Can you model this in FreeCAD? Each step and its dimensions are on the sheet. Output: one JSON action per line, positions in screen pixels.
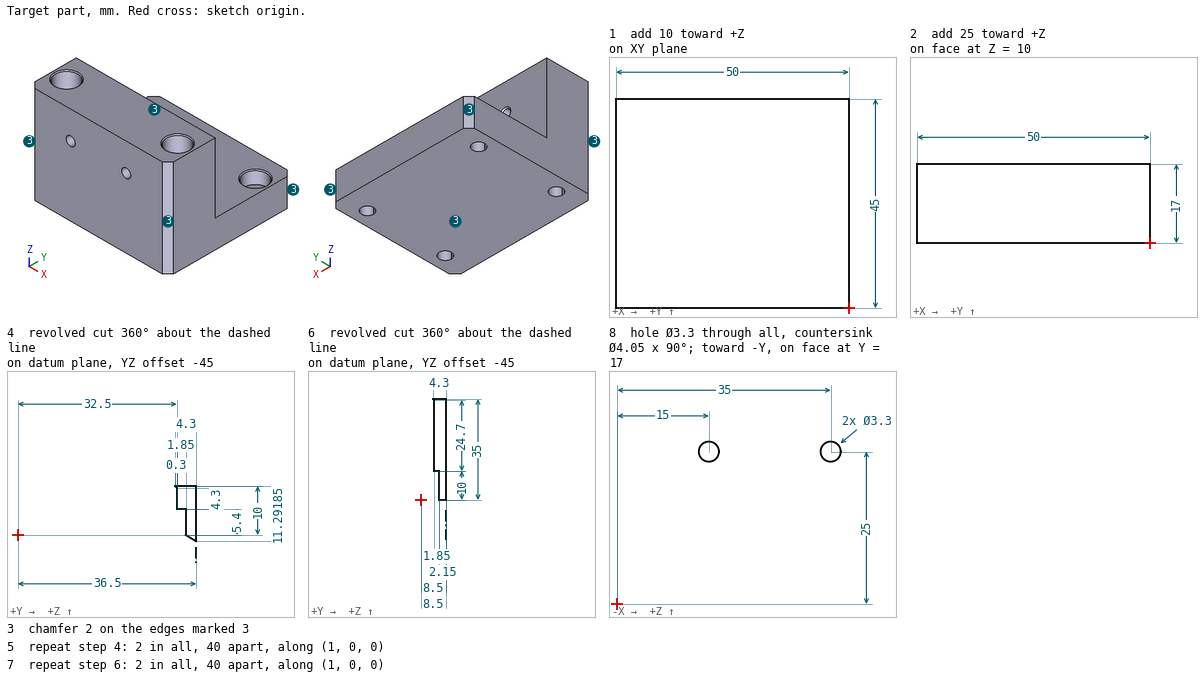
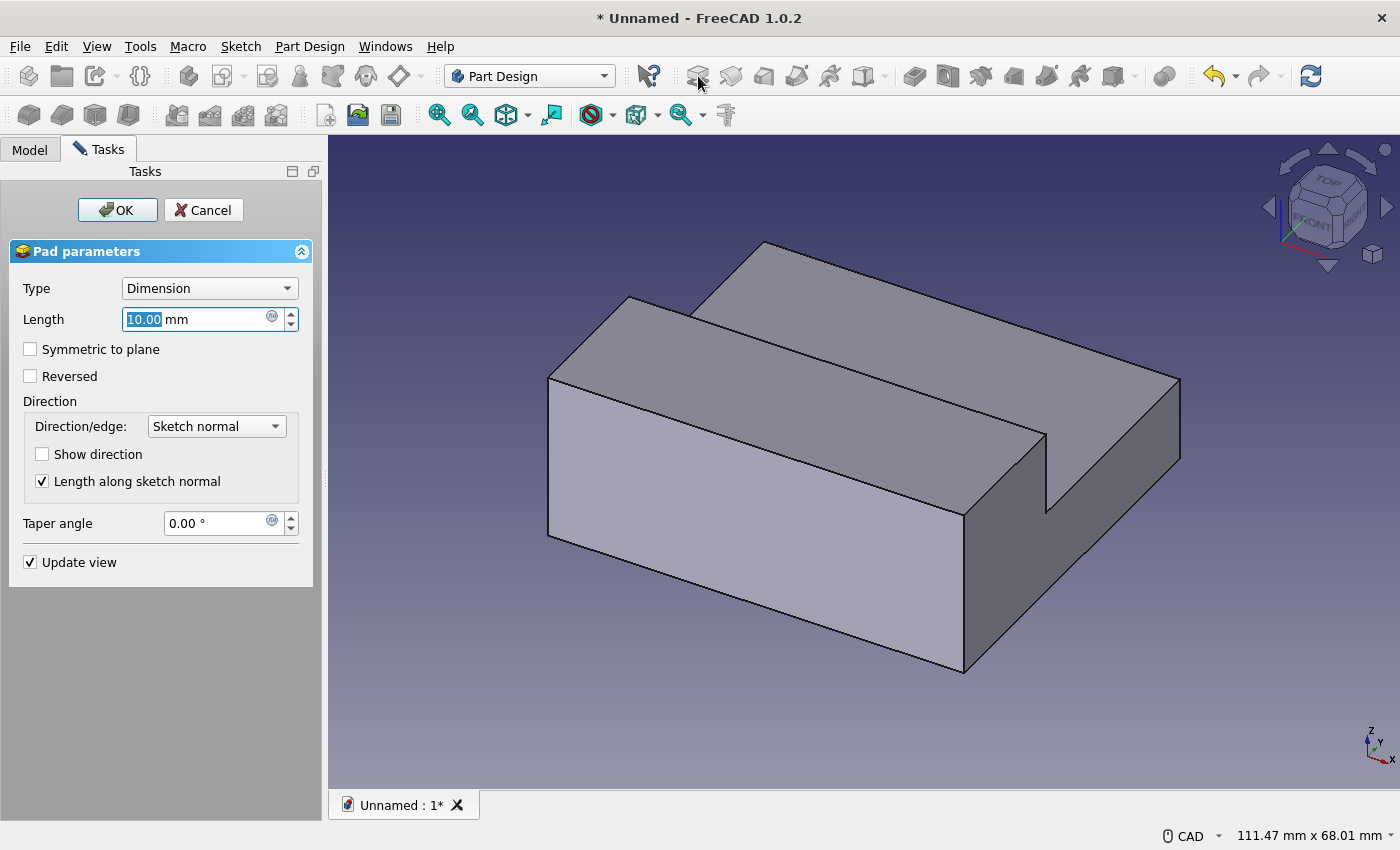
{"action": "type", "text": "25"}
{"action": "key", "text": "Tab"}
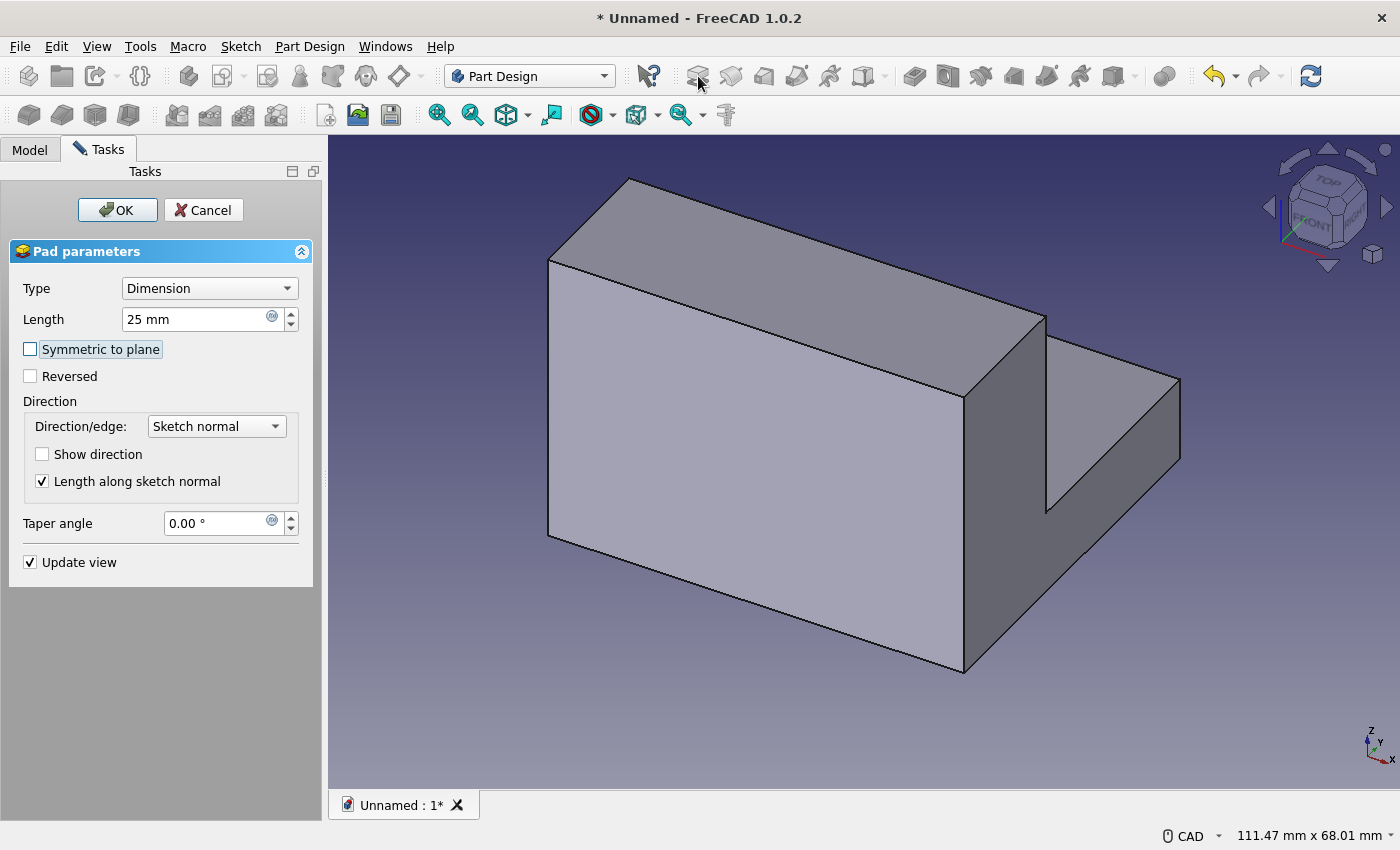
{"action": "left_click", "coordinate": [118, 210]}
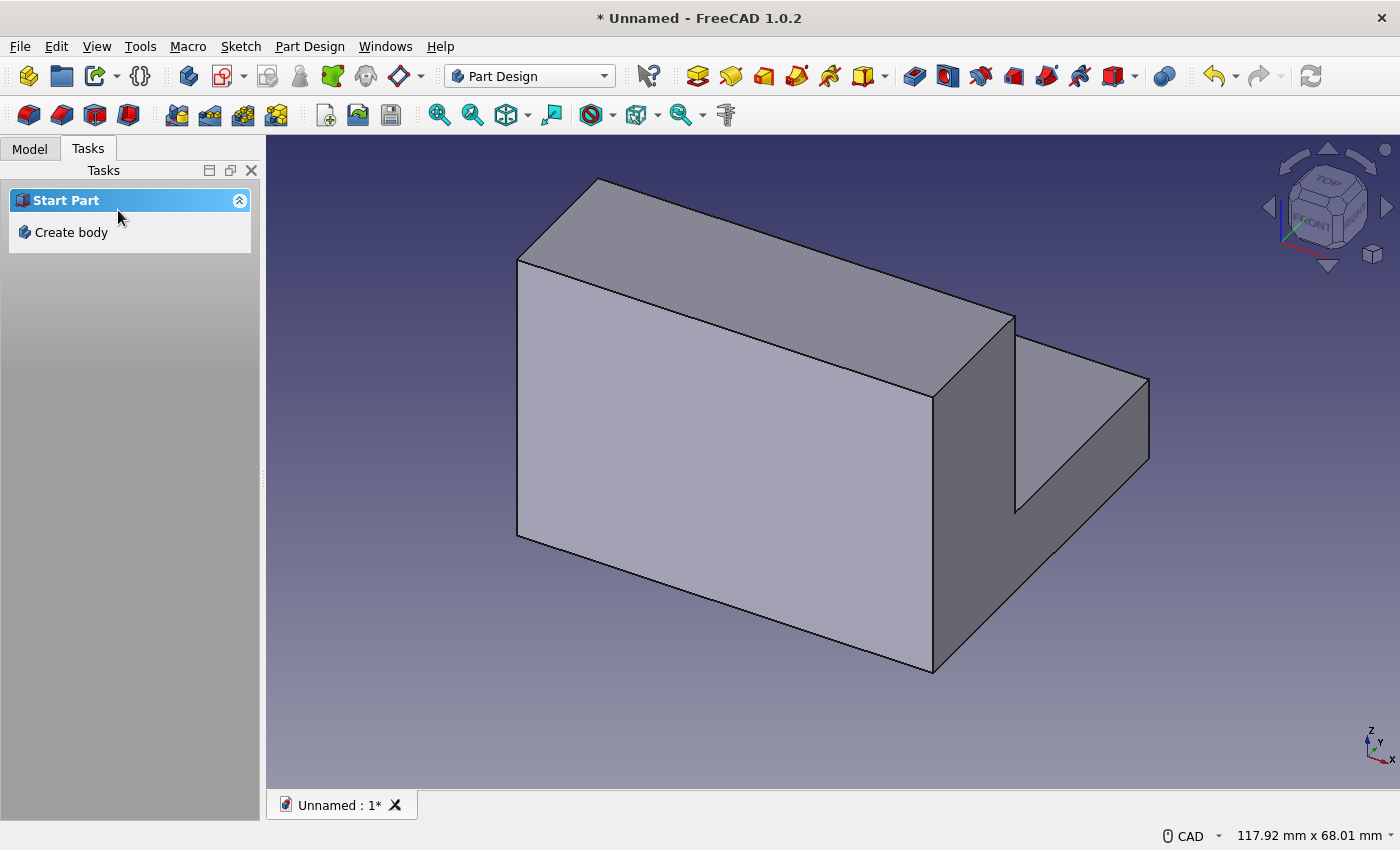
{"action": "key", "text": "v f"}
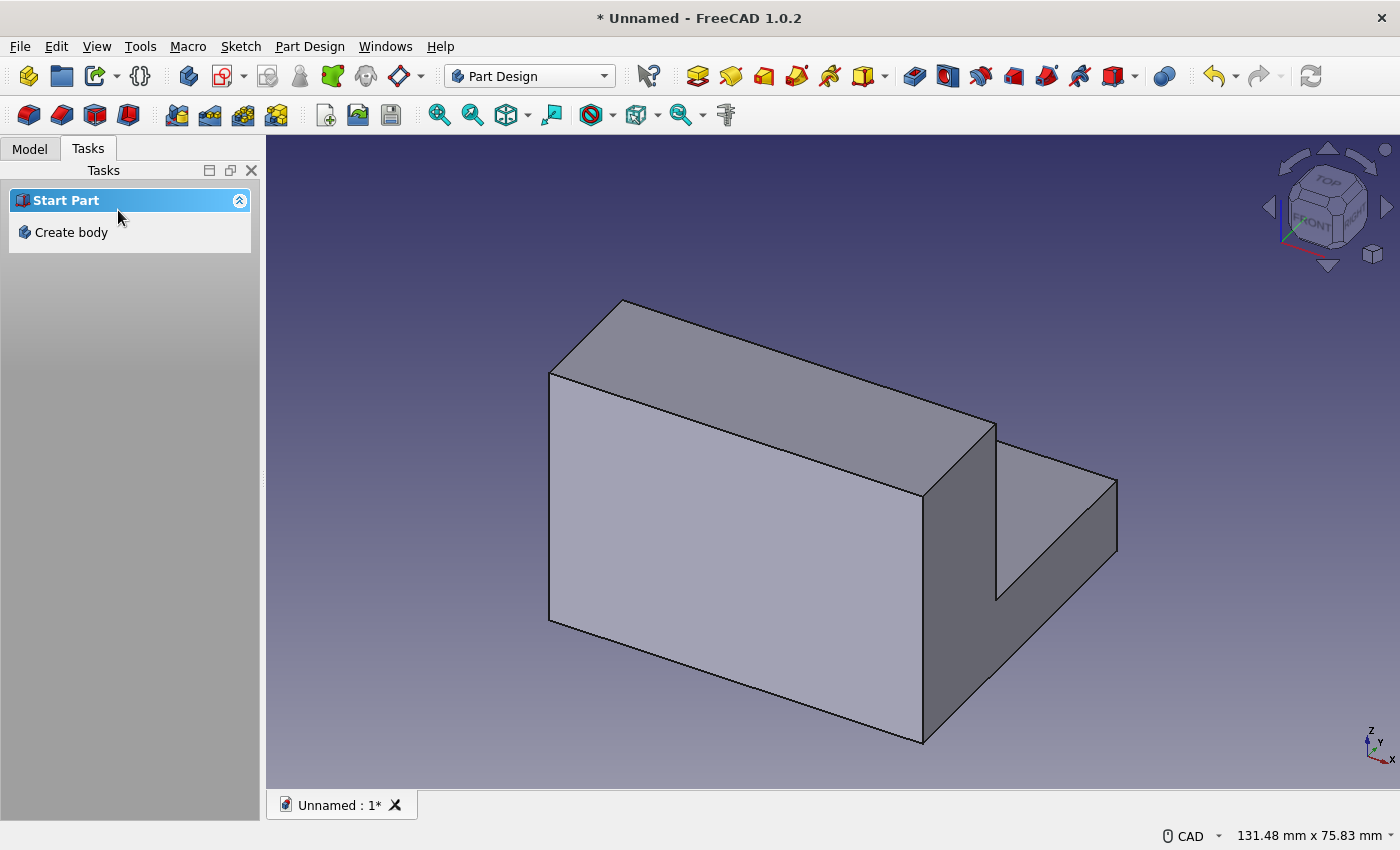
{"action": "left_click", "coordinate": [923, 619]}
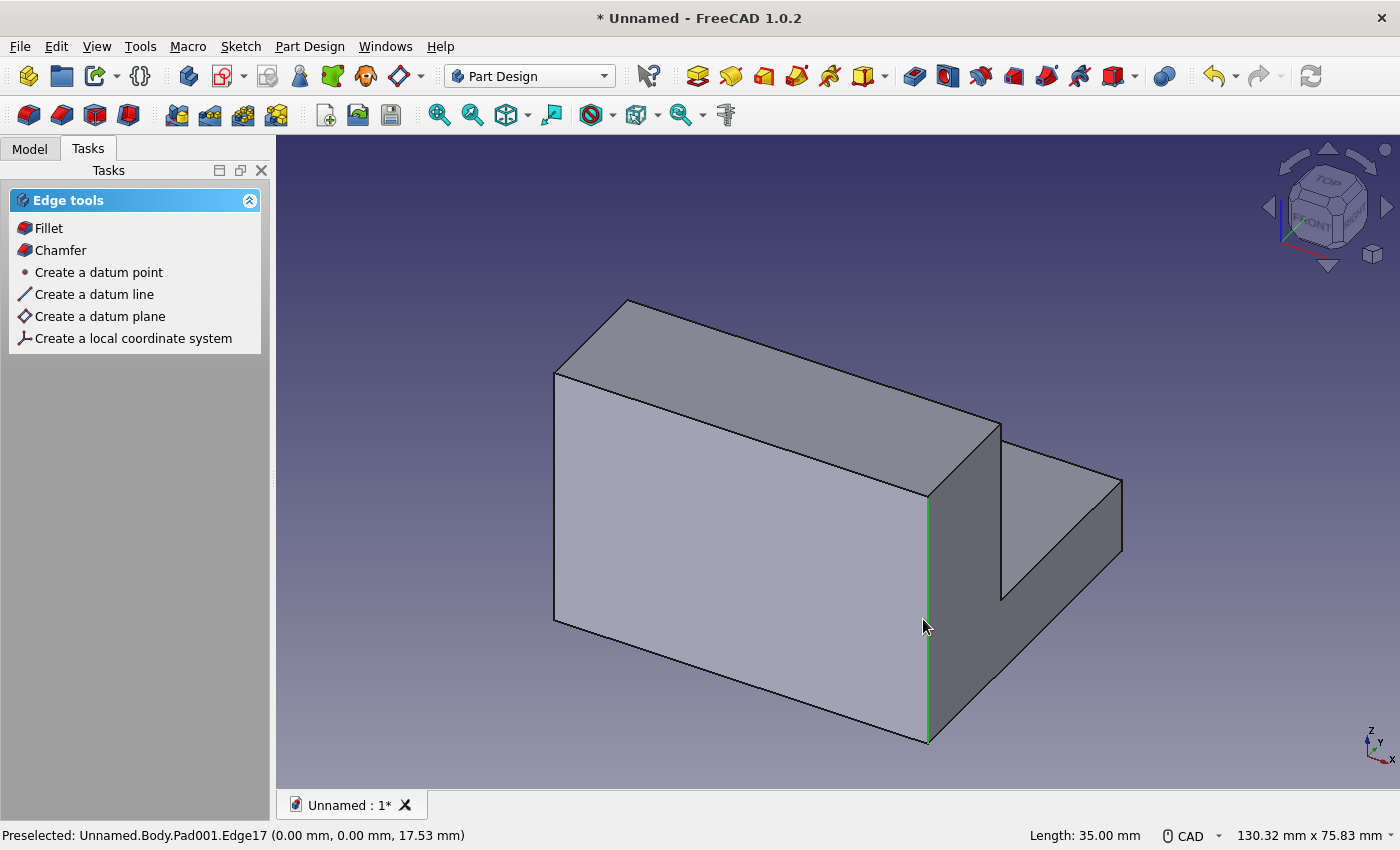
{"action": "key", "text": "0"}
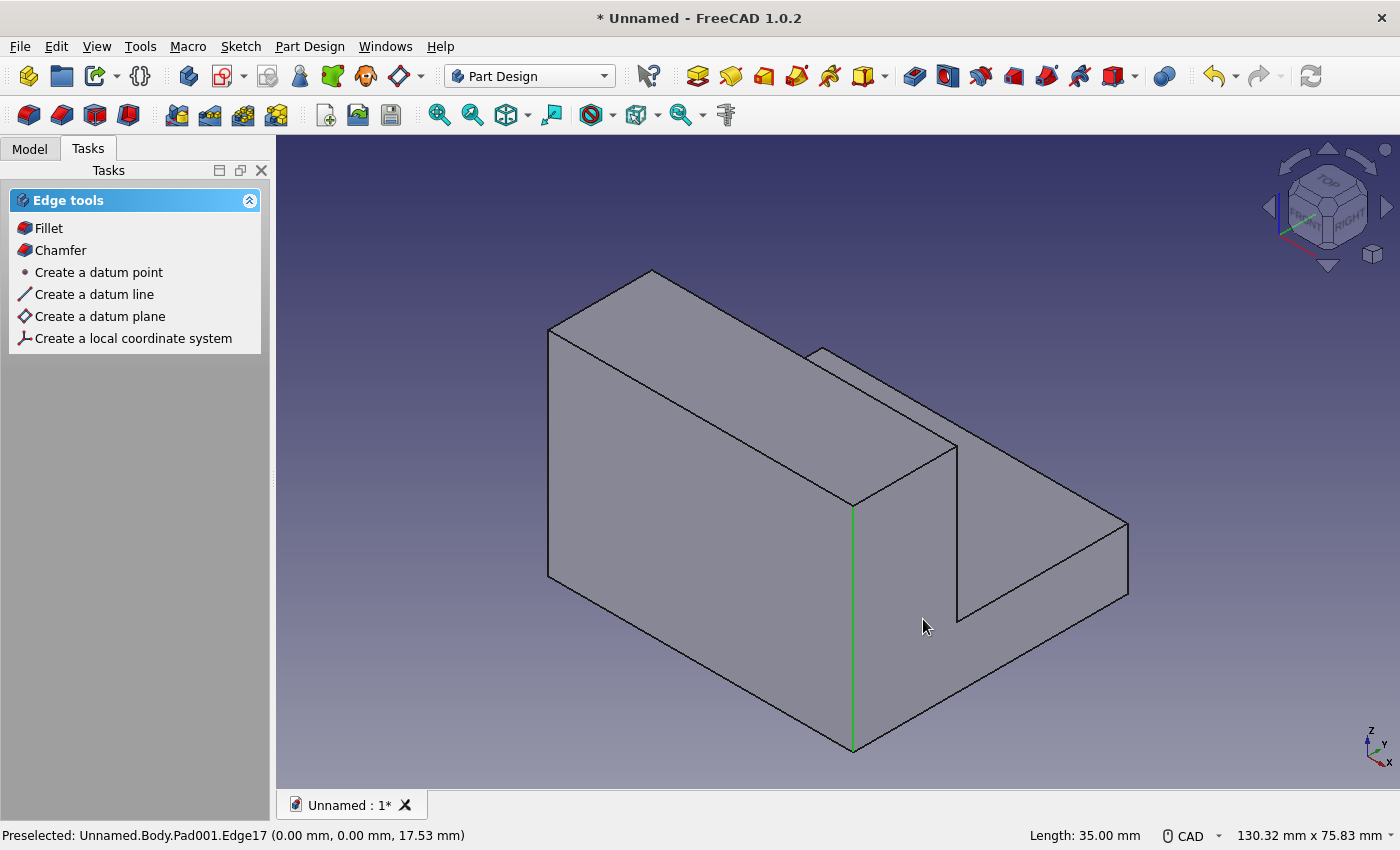
{"action": "key", "text": "2"}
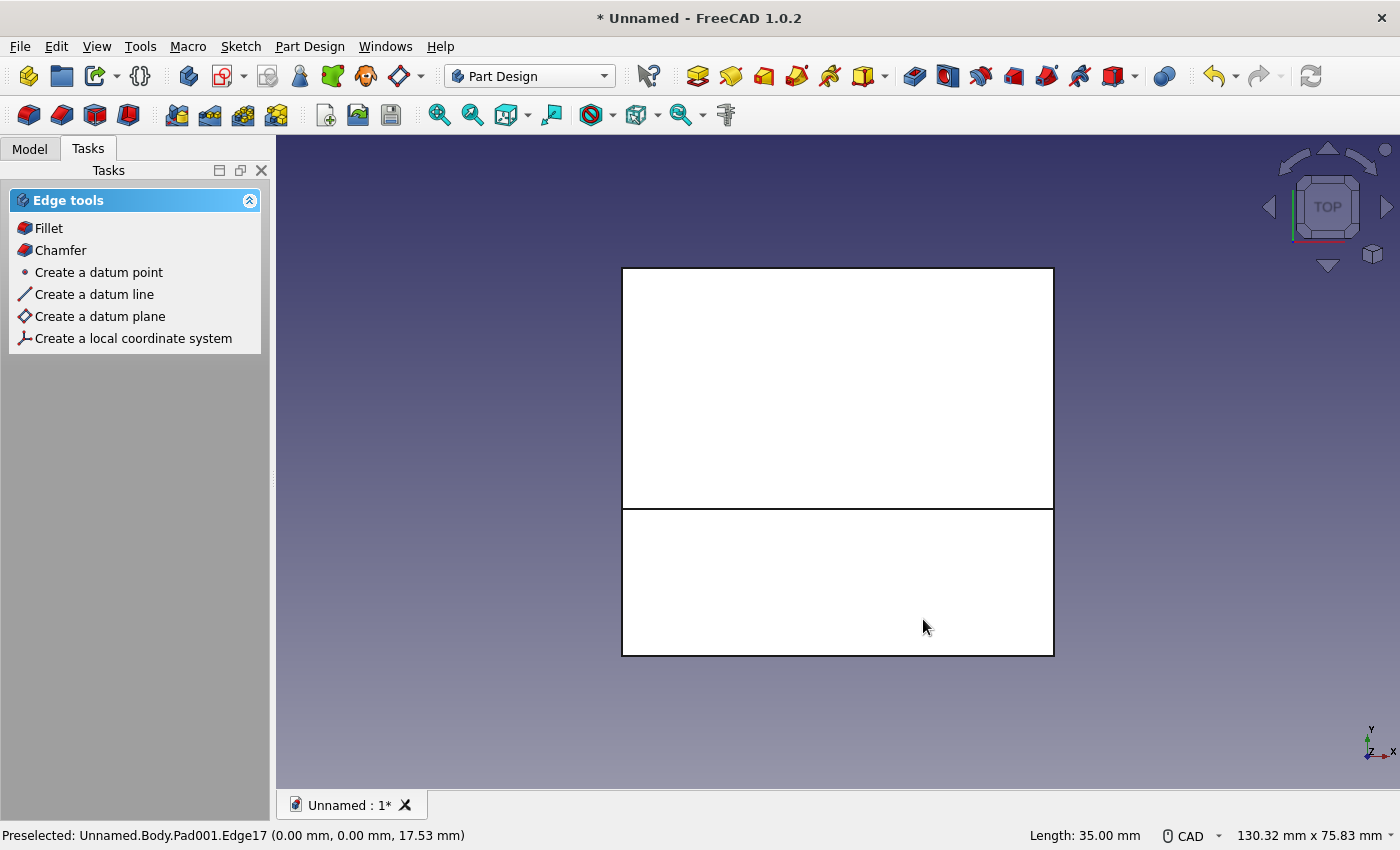
{"action": "key", "text": "1"}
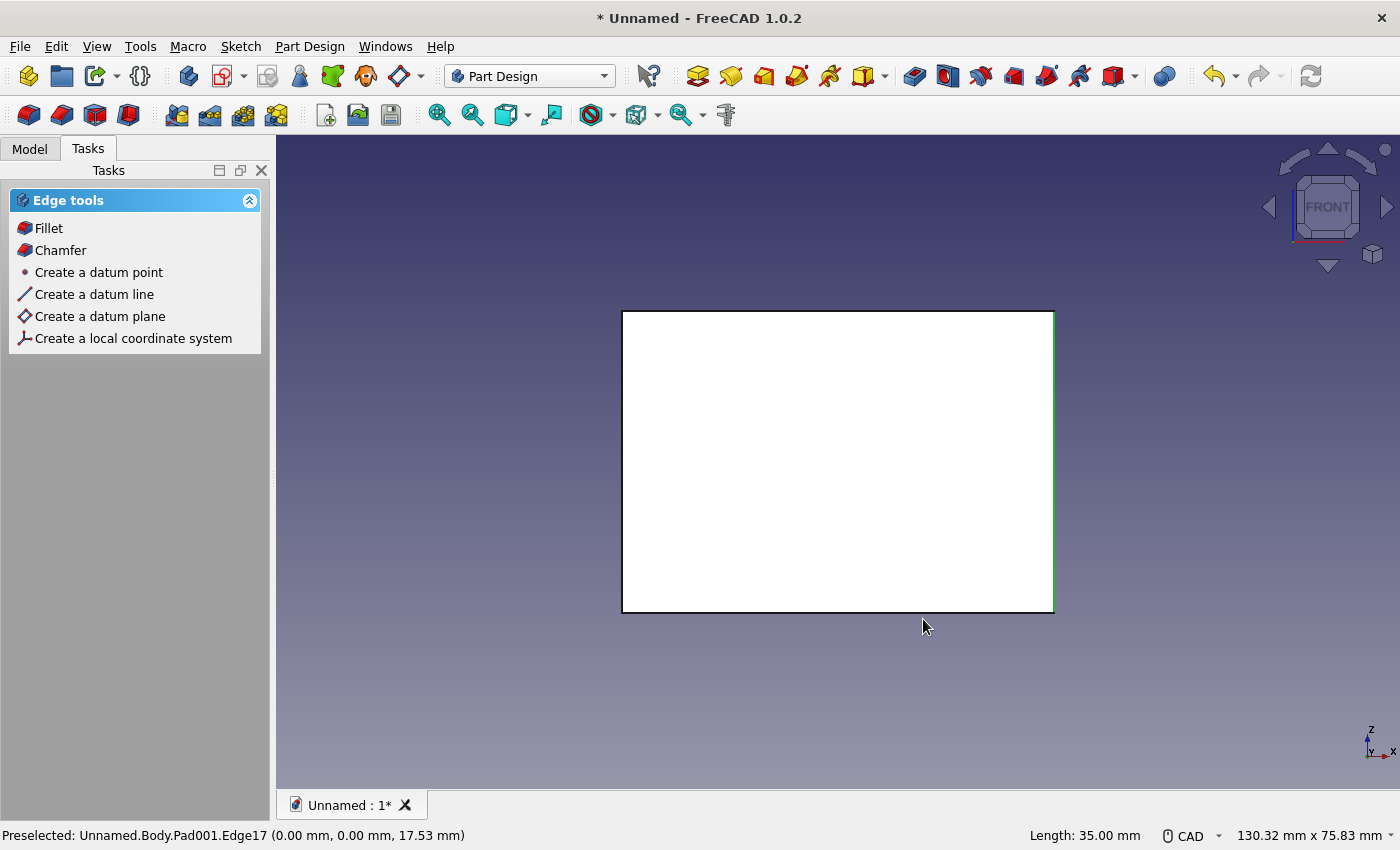
{"action": "left_click", "coordinate": [622, 461], "text": "ctrl"}